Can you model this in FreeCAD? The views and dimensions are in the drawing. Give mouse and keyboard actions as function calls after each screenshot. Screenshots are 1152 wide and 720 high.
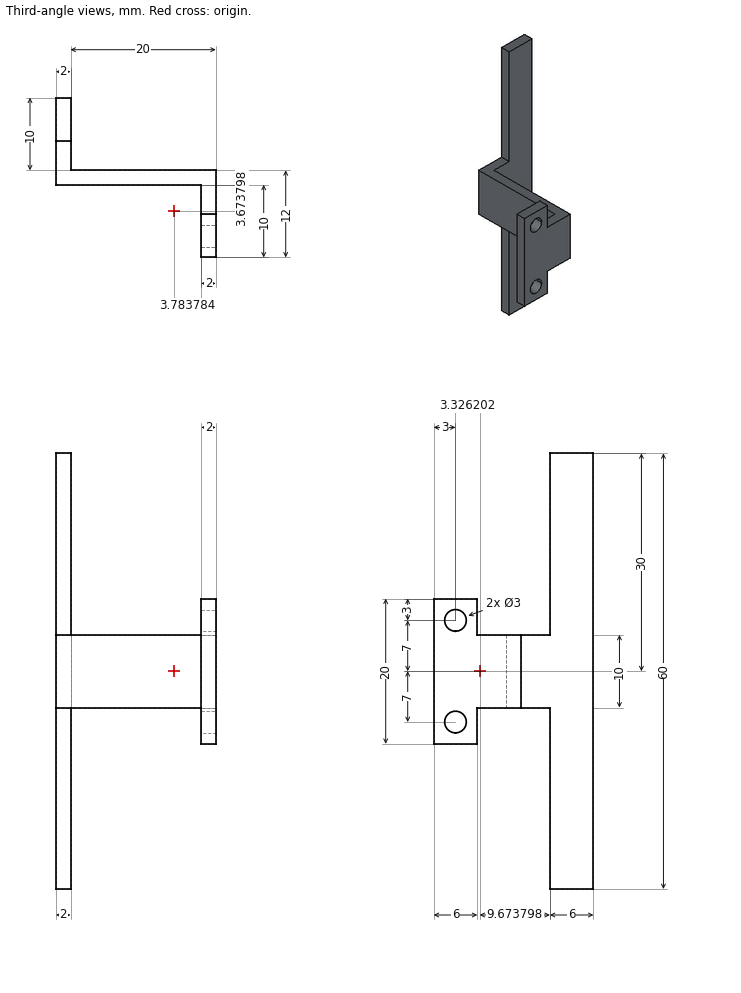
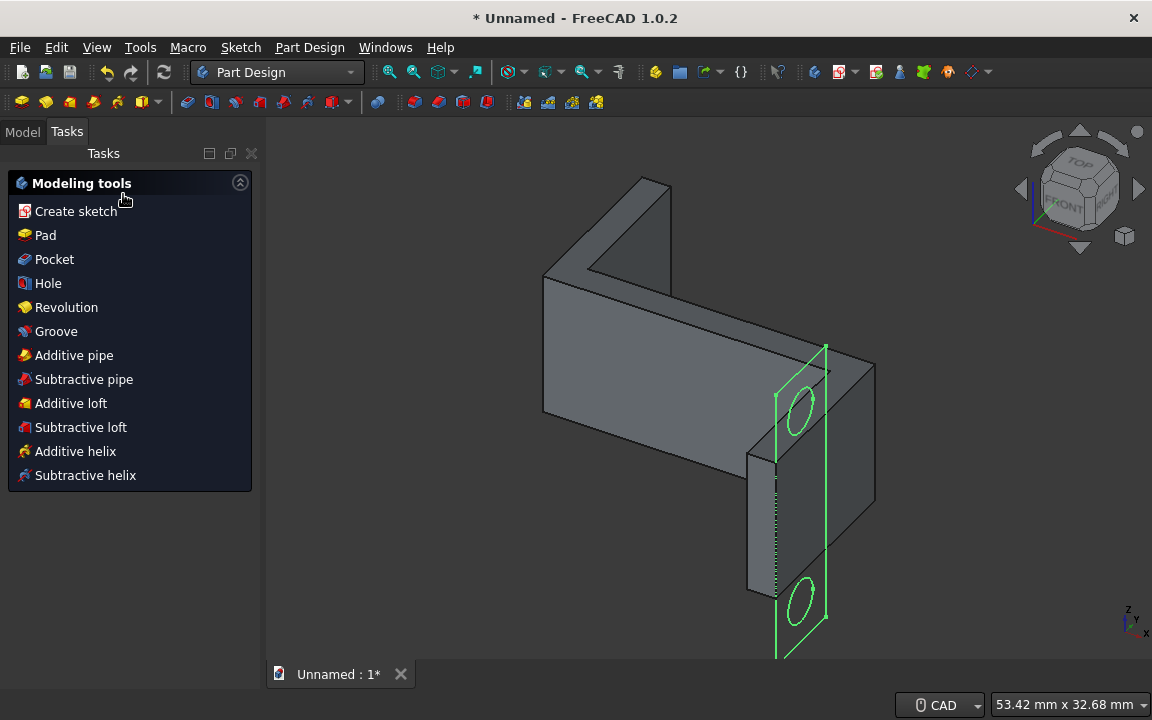
click(22, 102)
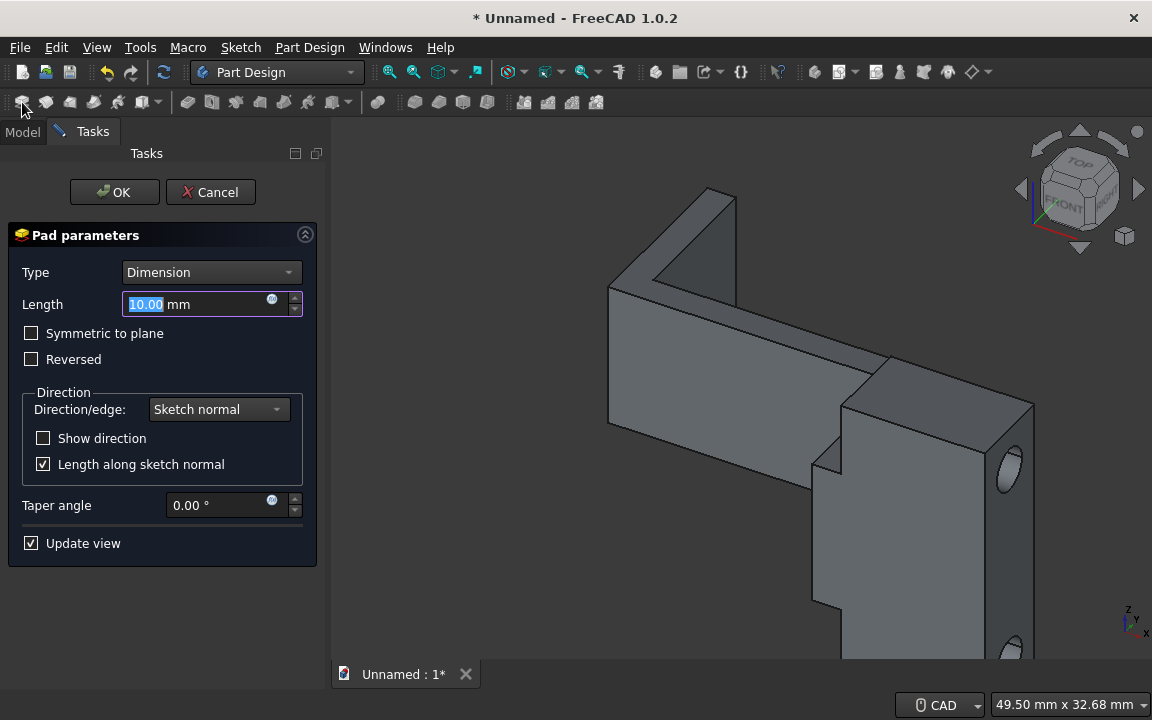
text(2)
key(Tab)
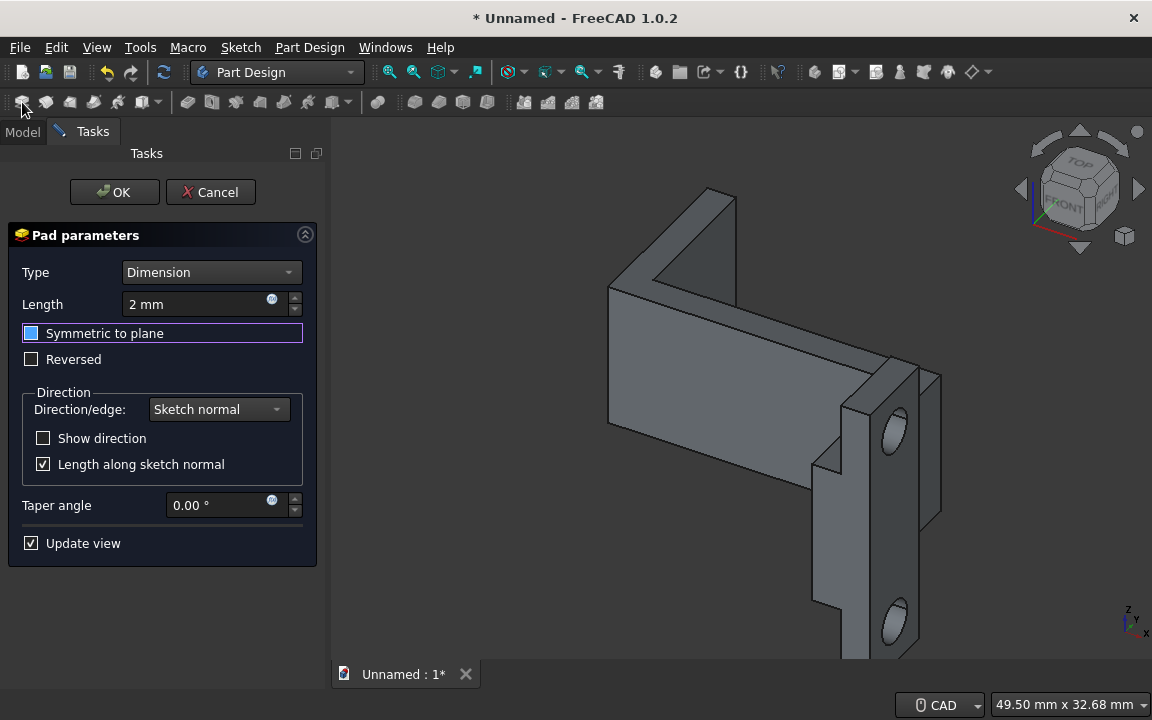
click(30, 359)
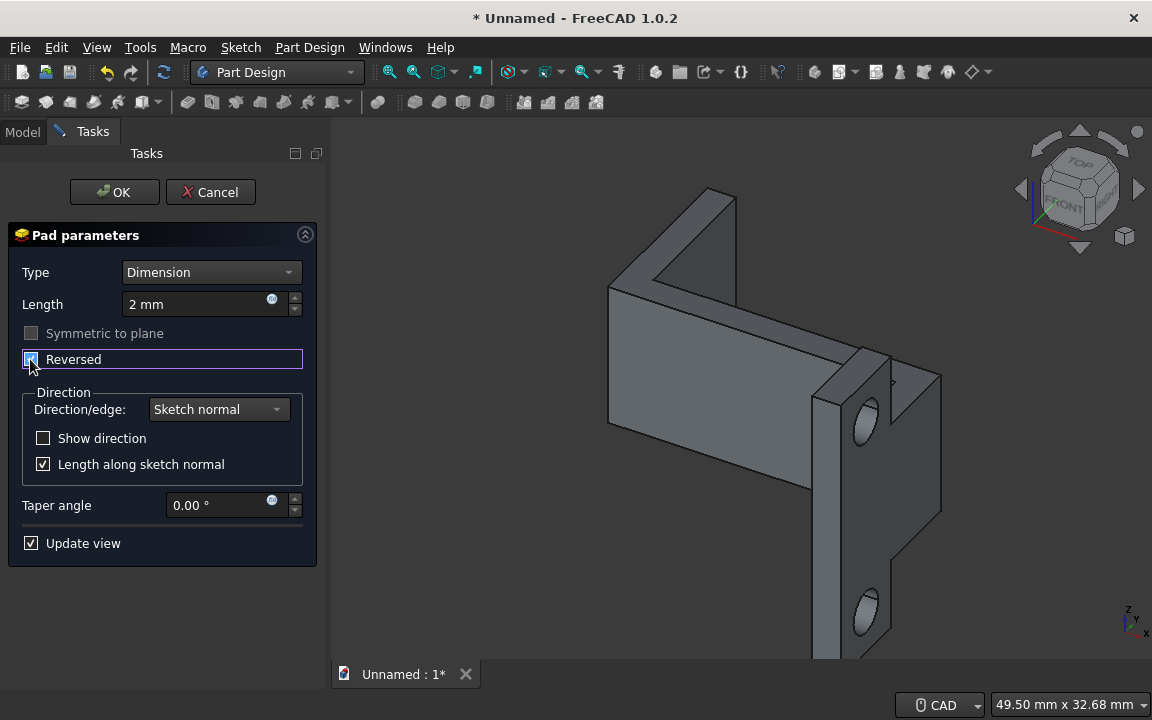
click(115, 192)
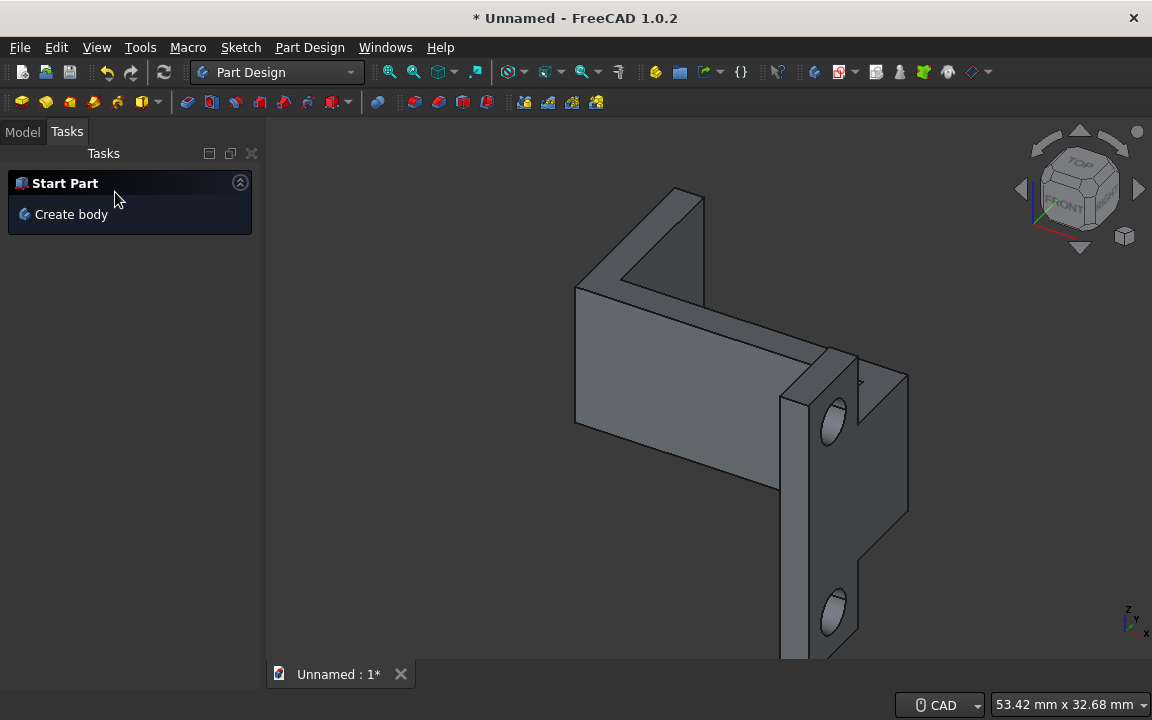
click(390, 72)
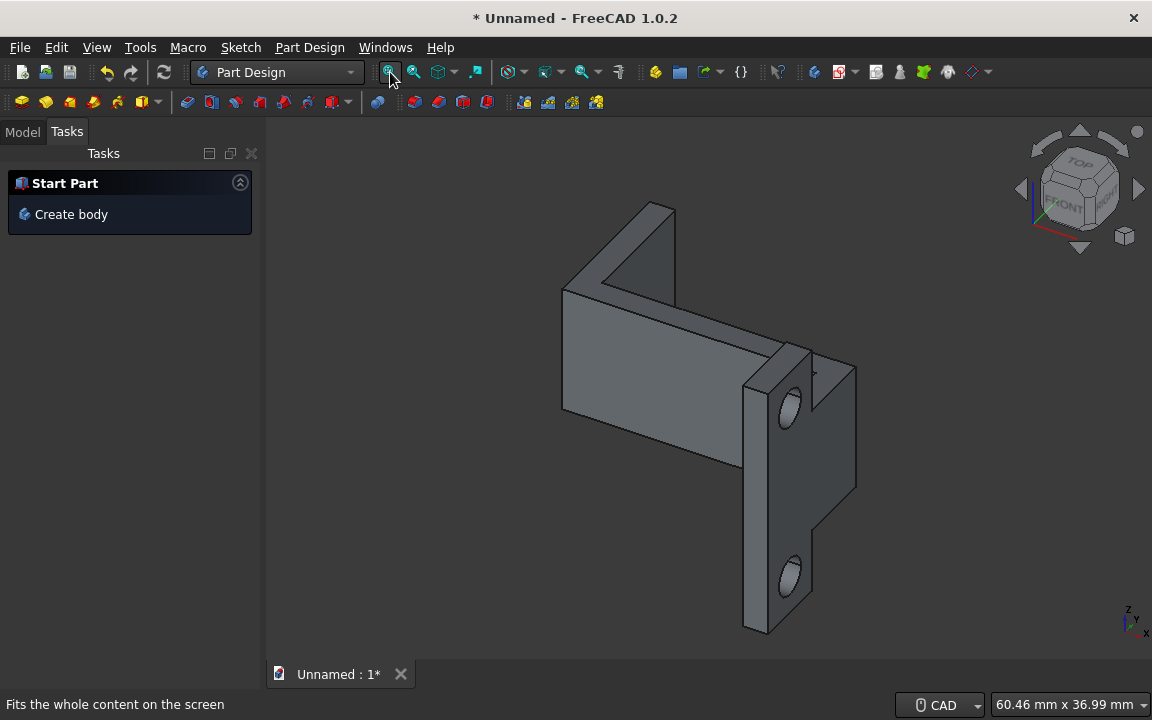
key(6)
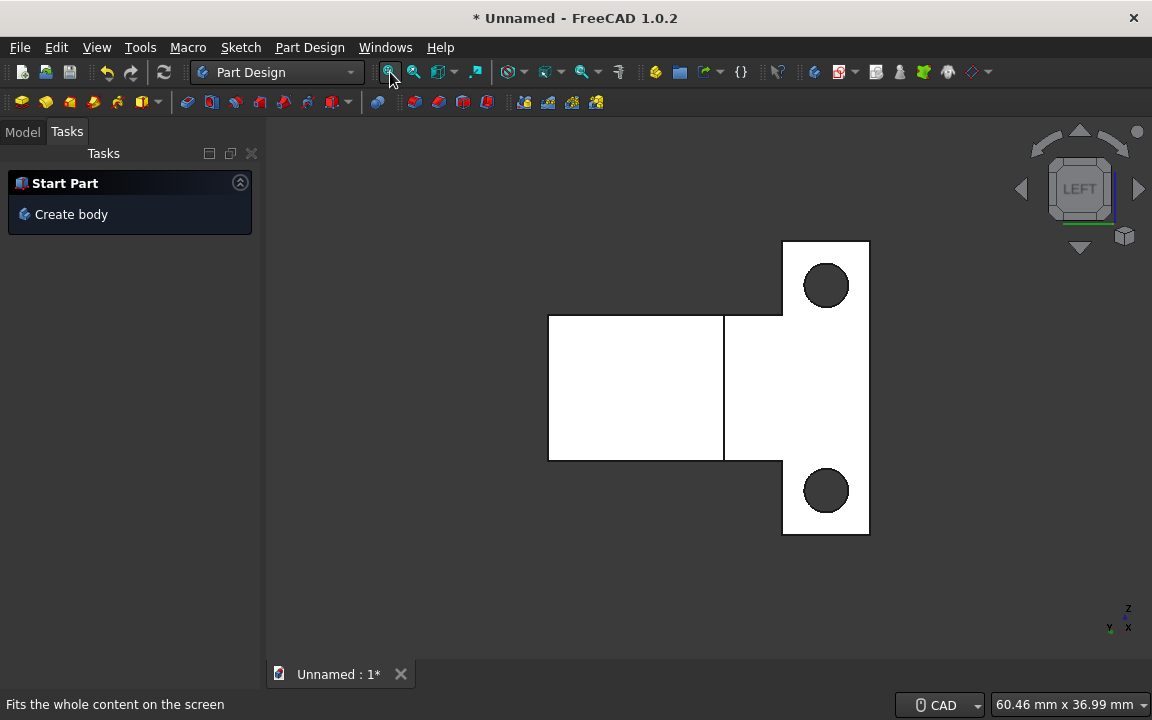
click(636, 387)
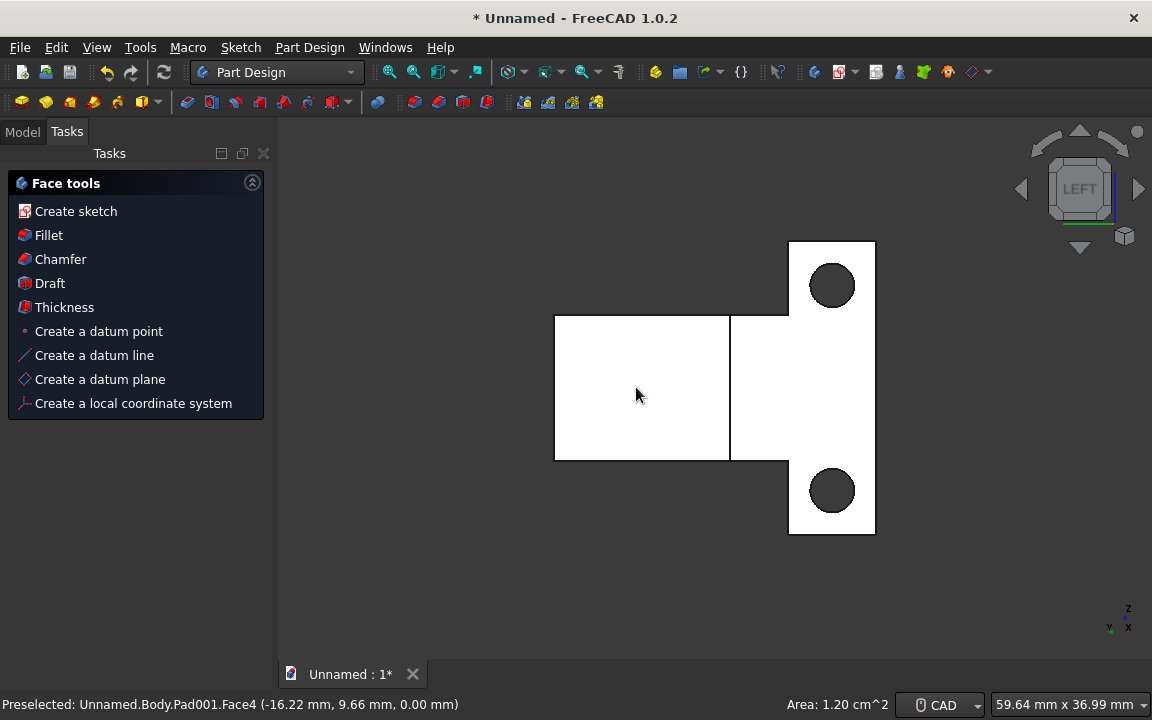
click(840, 72)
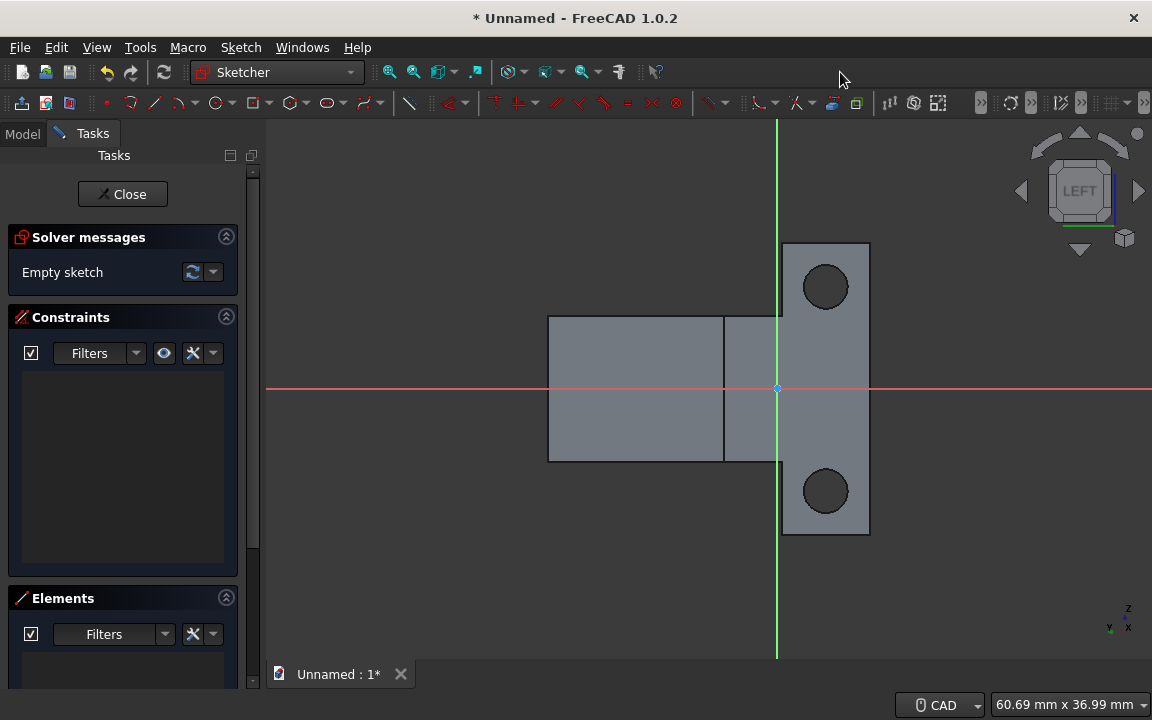
scroll(628, 389, down, 5)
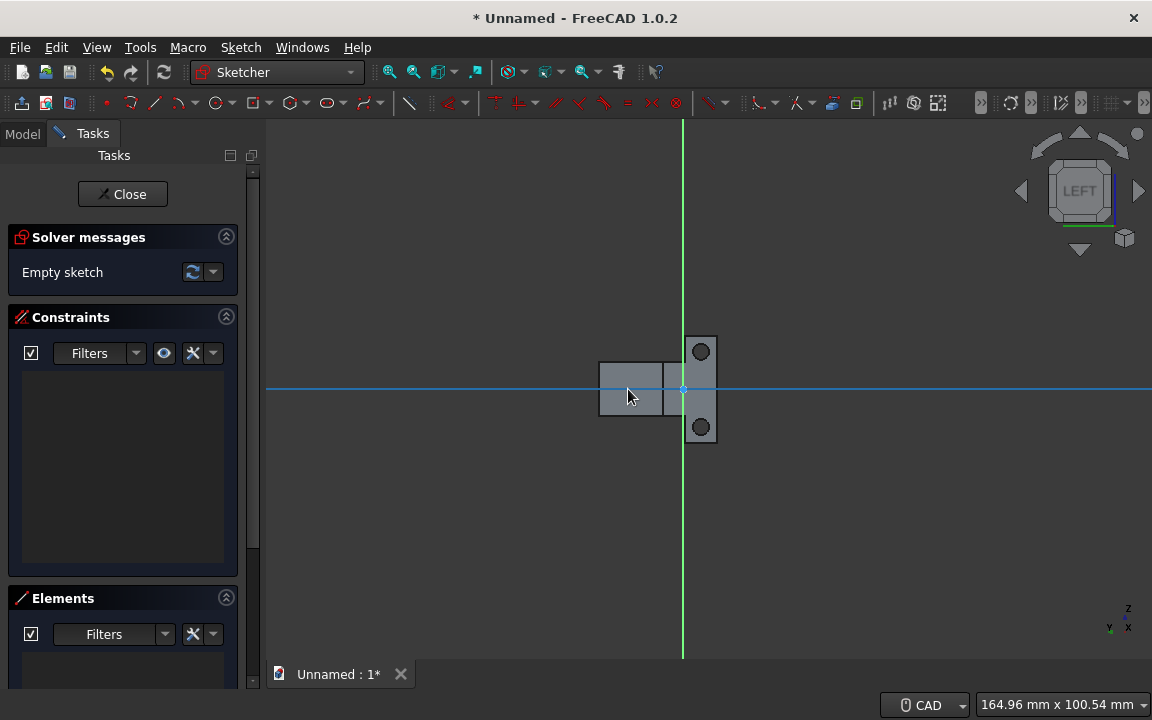
key(g)
key(r)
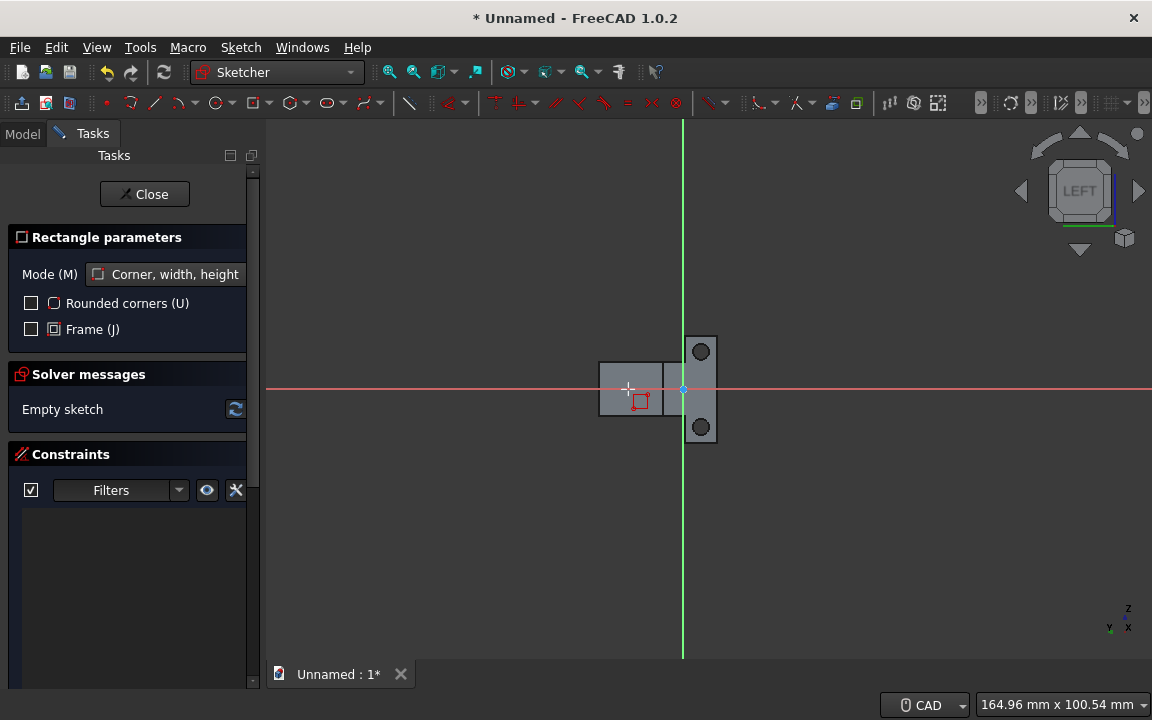
click(599, 228)
click(631, 550)
key(Escape)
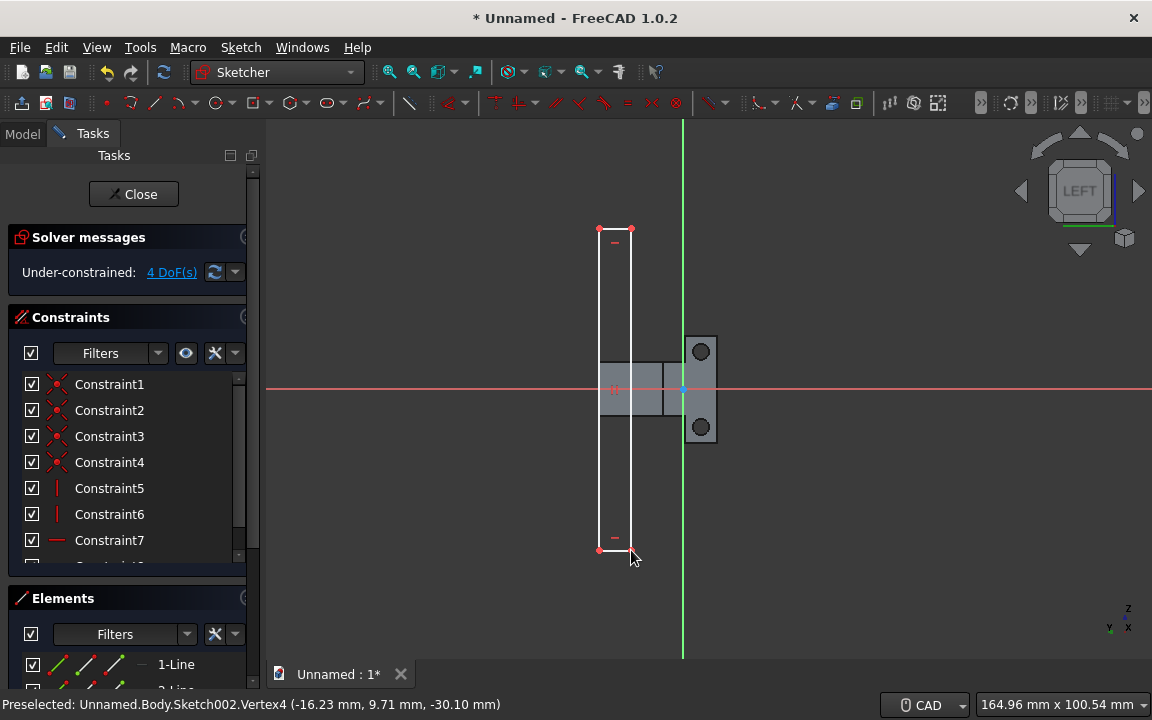
key(d)